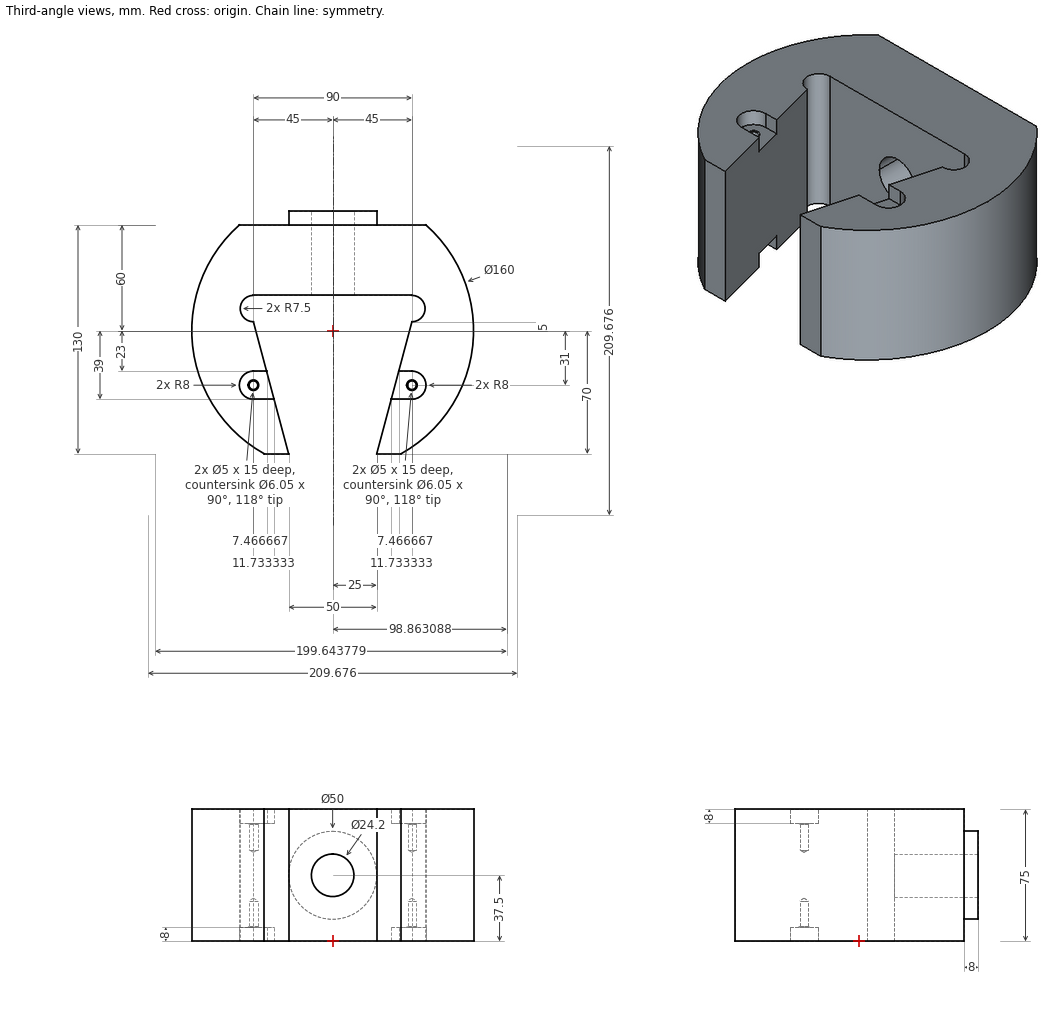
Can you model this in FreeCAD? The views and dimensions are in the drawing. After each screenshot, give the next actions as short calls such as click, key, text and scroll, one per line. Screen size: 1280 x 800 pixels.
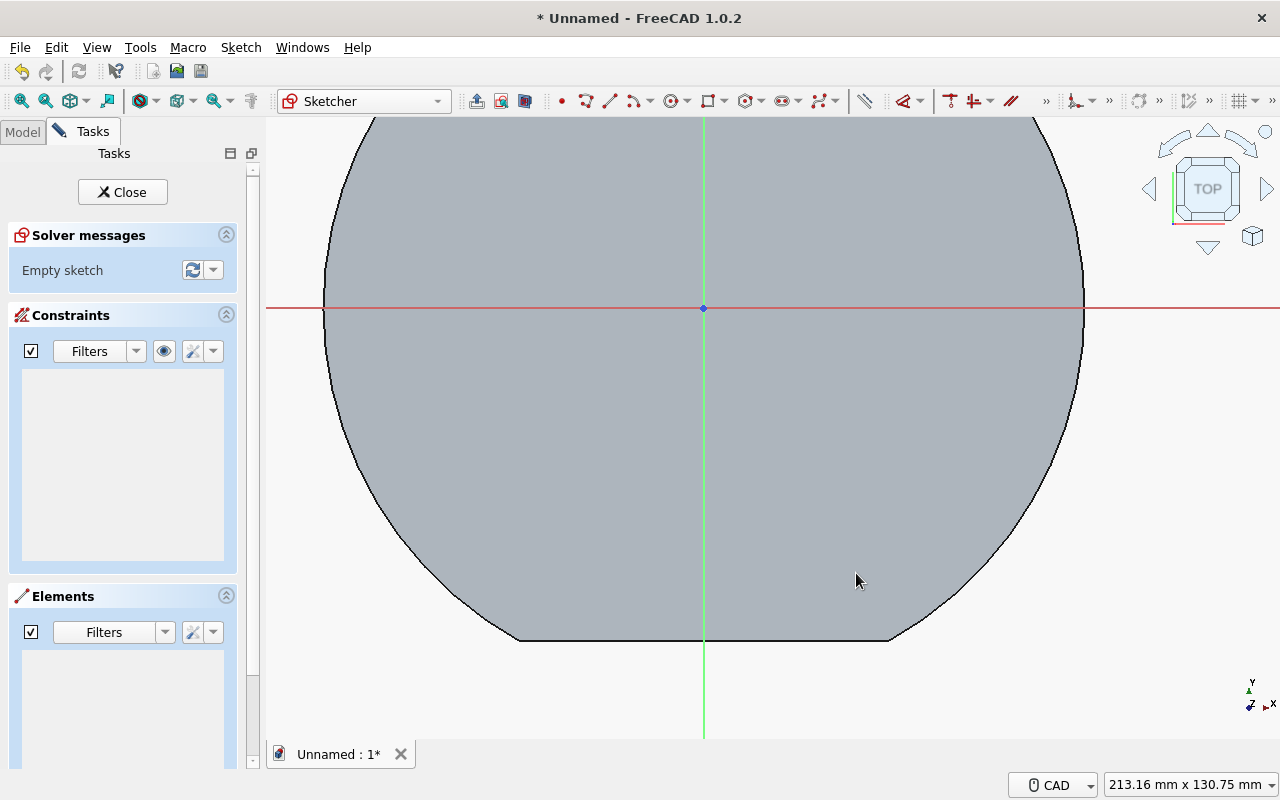
key(g)
key(m)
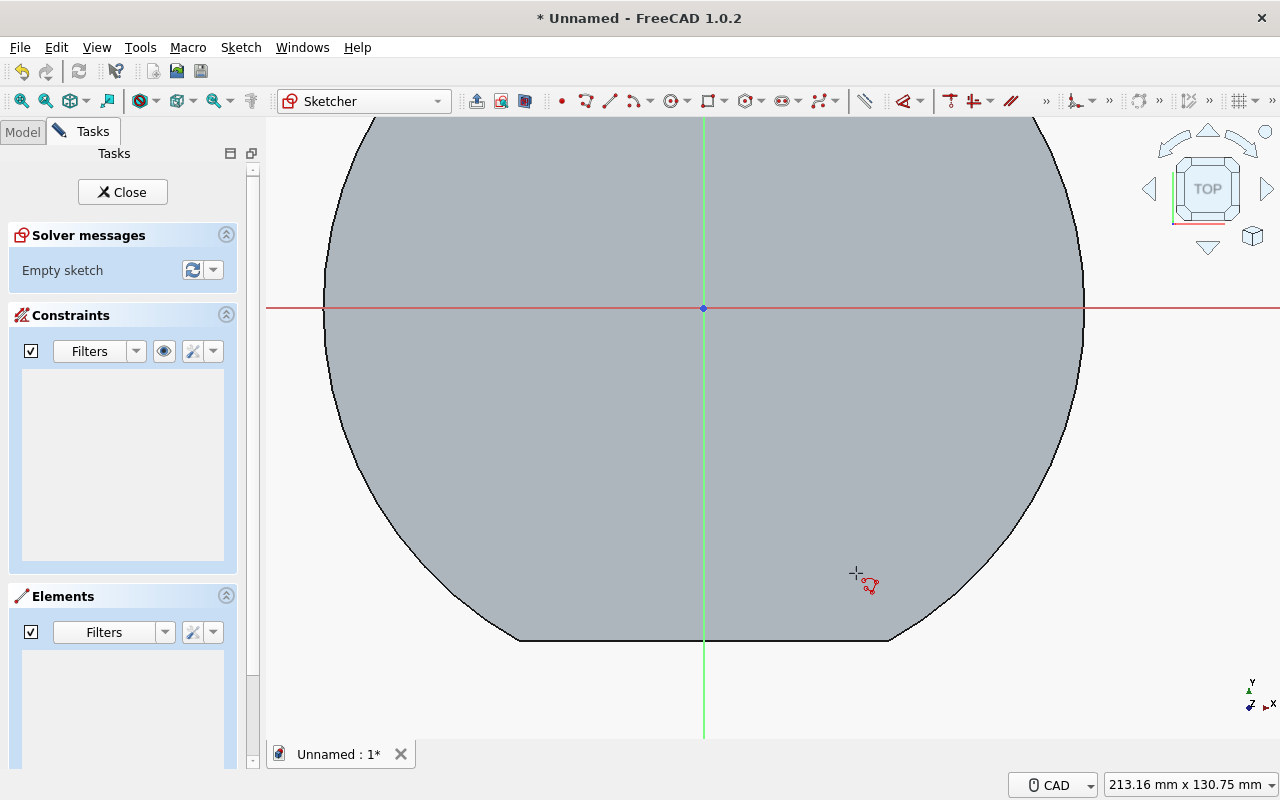
click(918, 284)
click(823, 641)
click(585, 641)
click(490, 284)
right_click(490, 284)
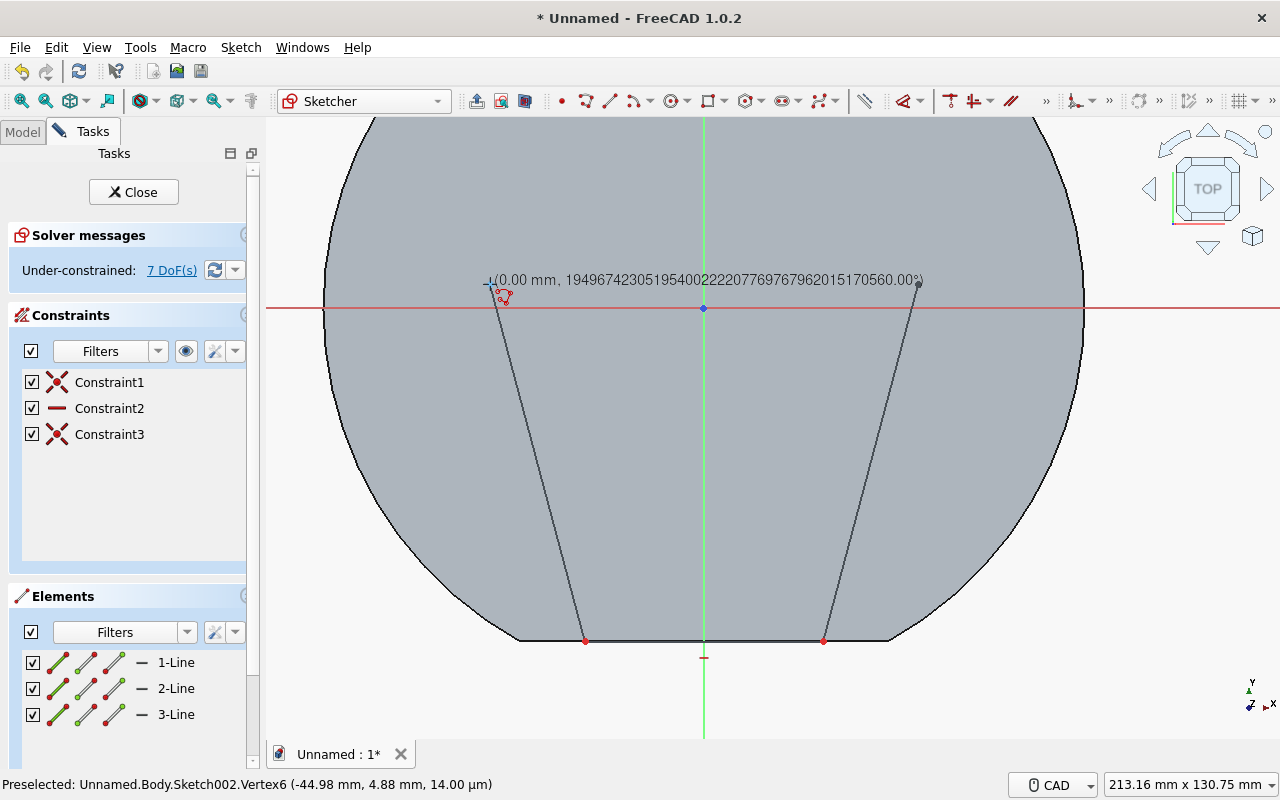
key(g)
key(l)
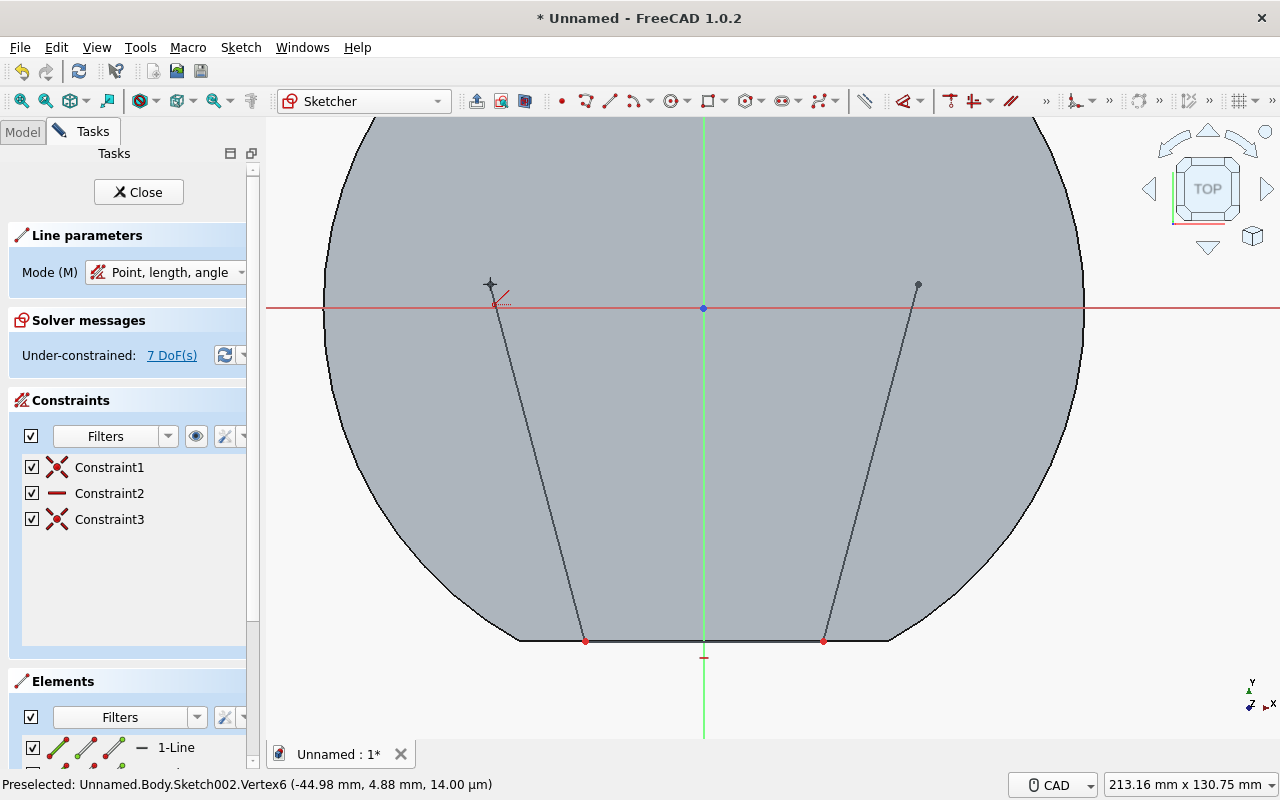
click(490, 213)
click(918, 213)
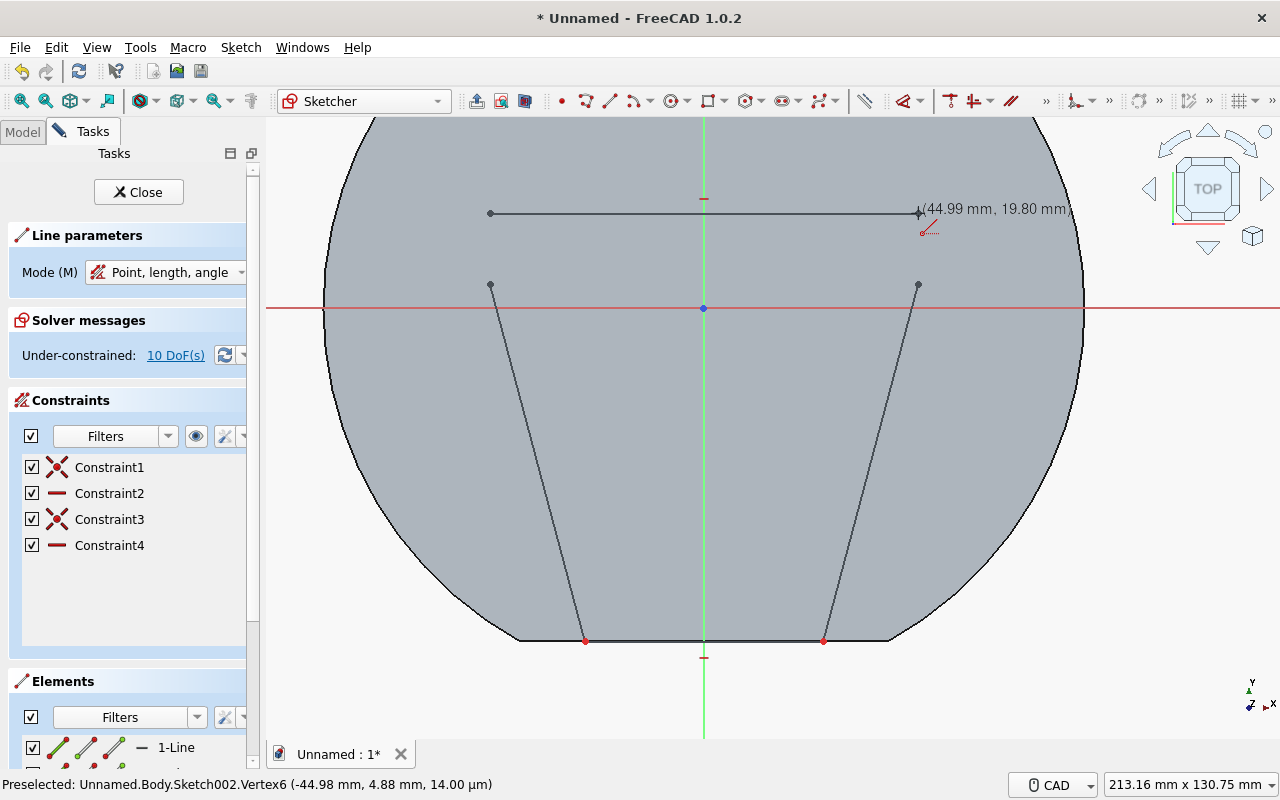
click(652, 102)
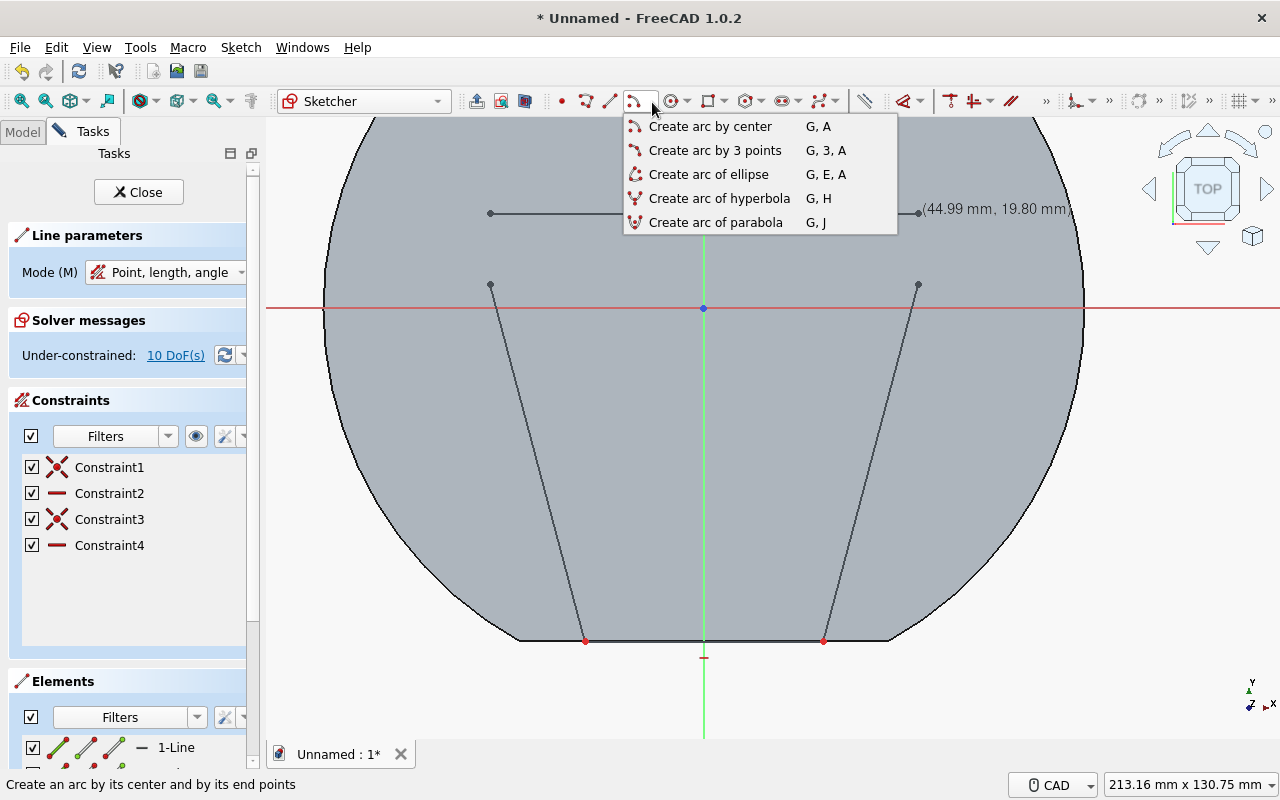
click(760, 150)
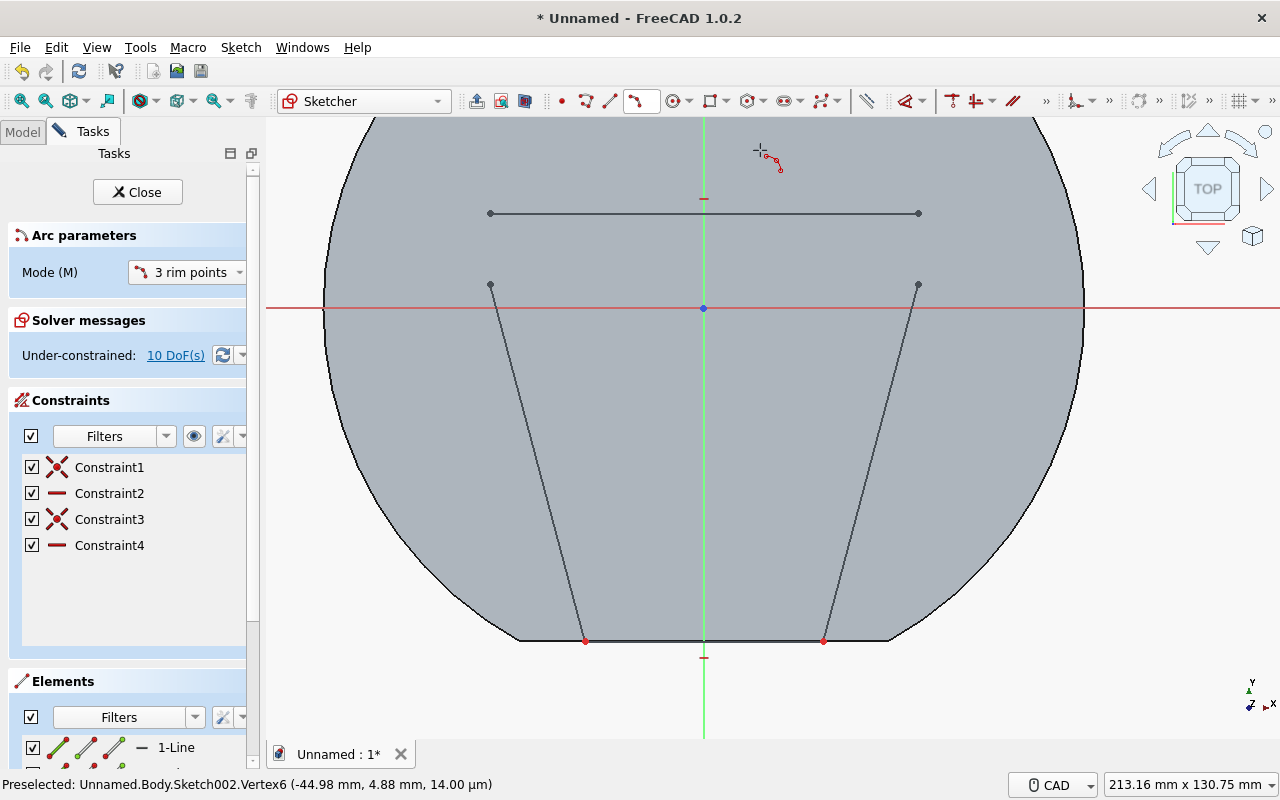
click(490, 285)
click(490, 214)
click(454, 249)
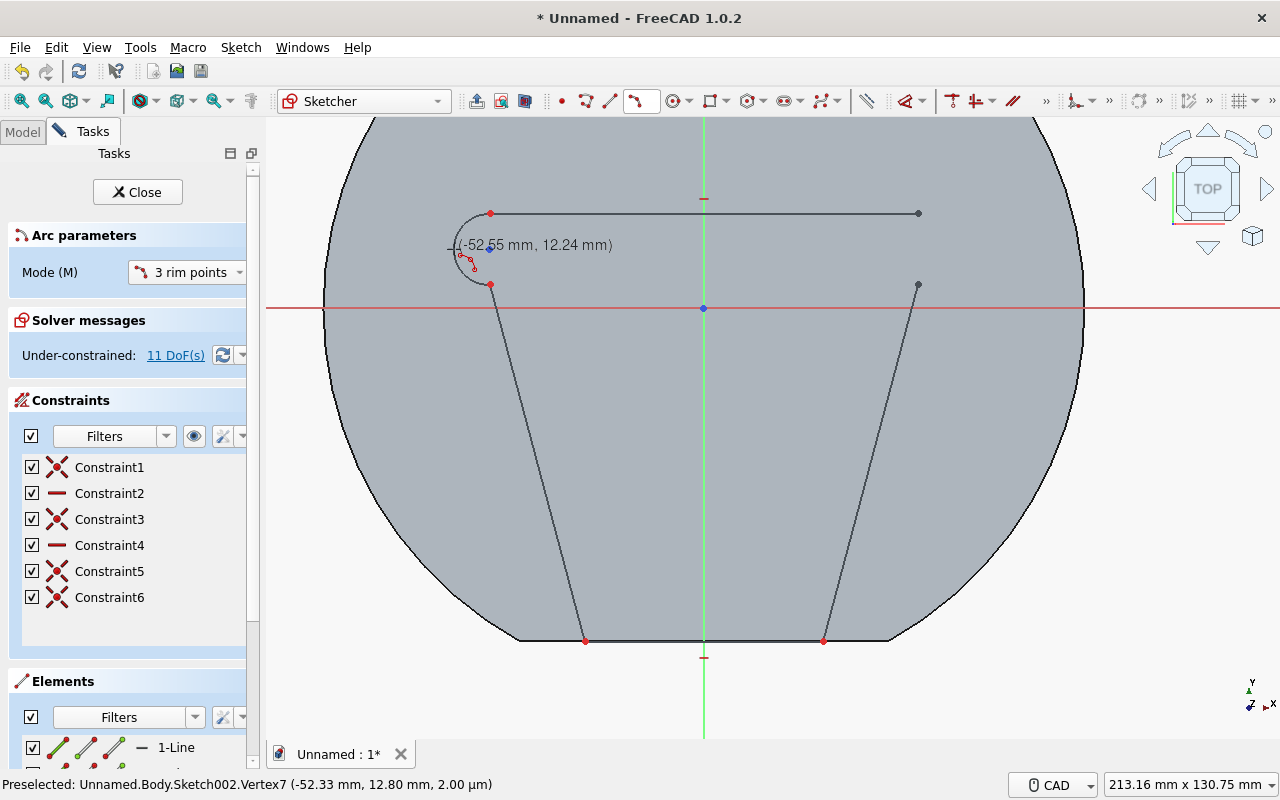
click(918, 214)
click(918, 285)
click(954, 249)
key(Escape)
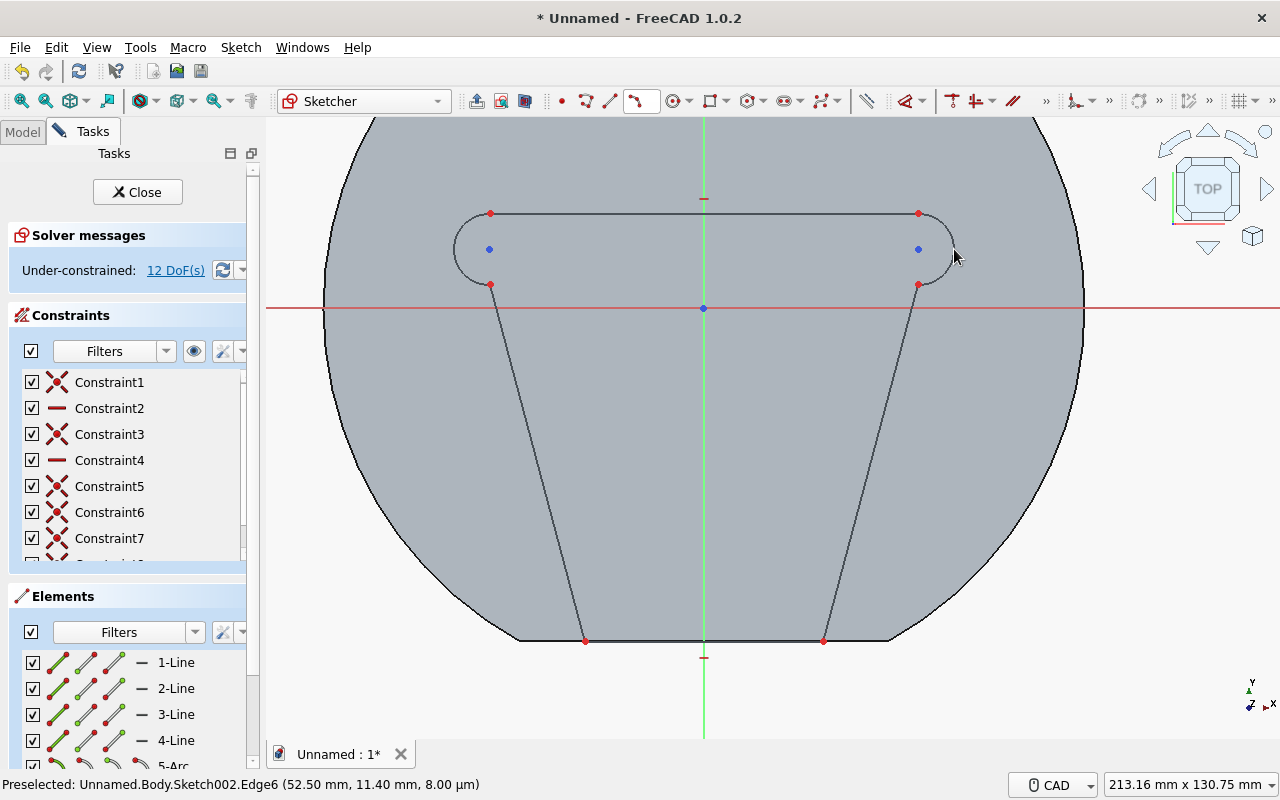
click(618, 214)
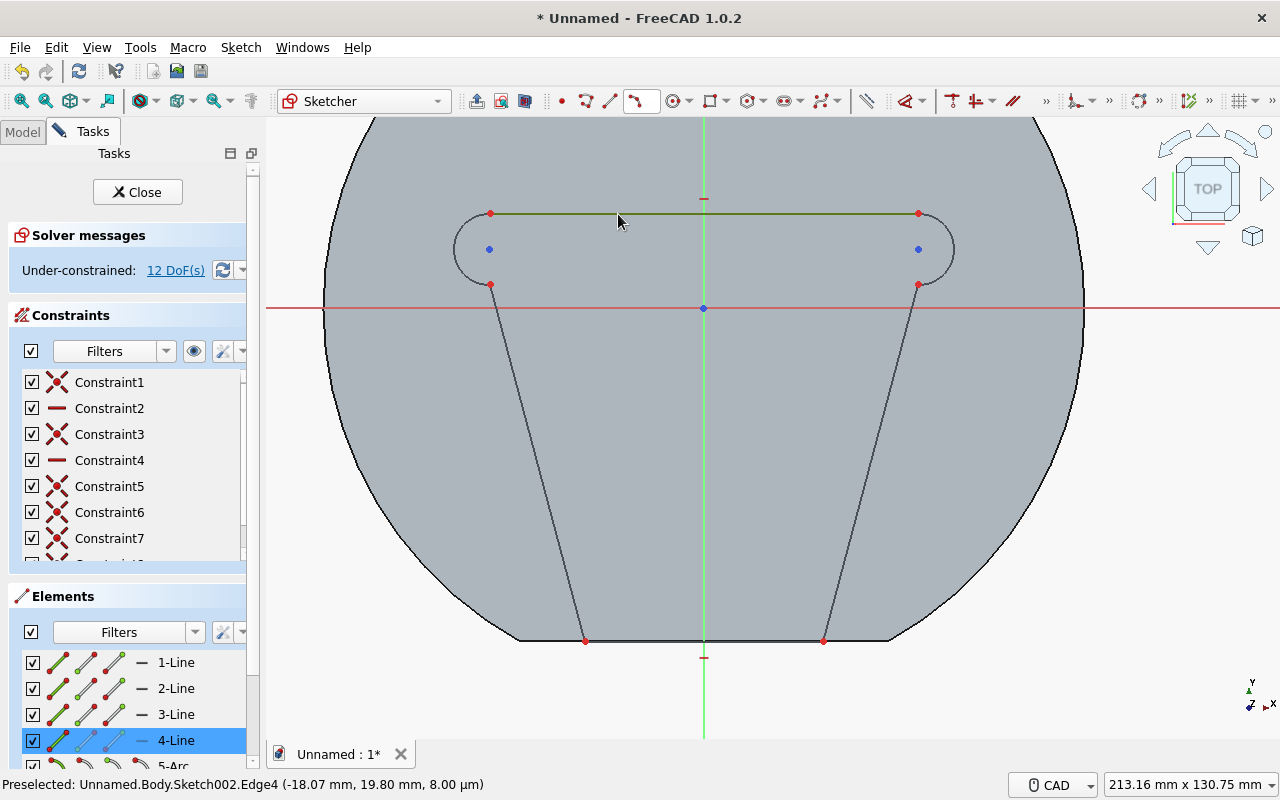
click(461, 228)